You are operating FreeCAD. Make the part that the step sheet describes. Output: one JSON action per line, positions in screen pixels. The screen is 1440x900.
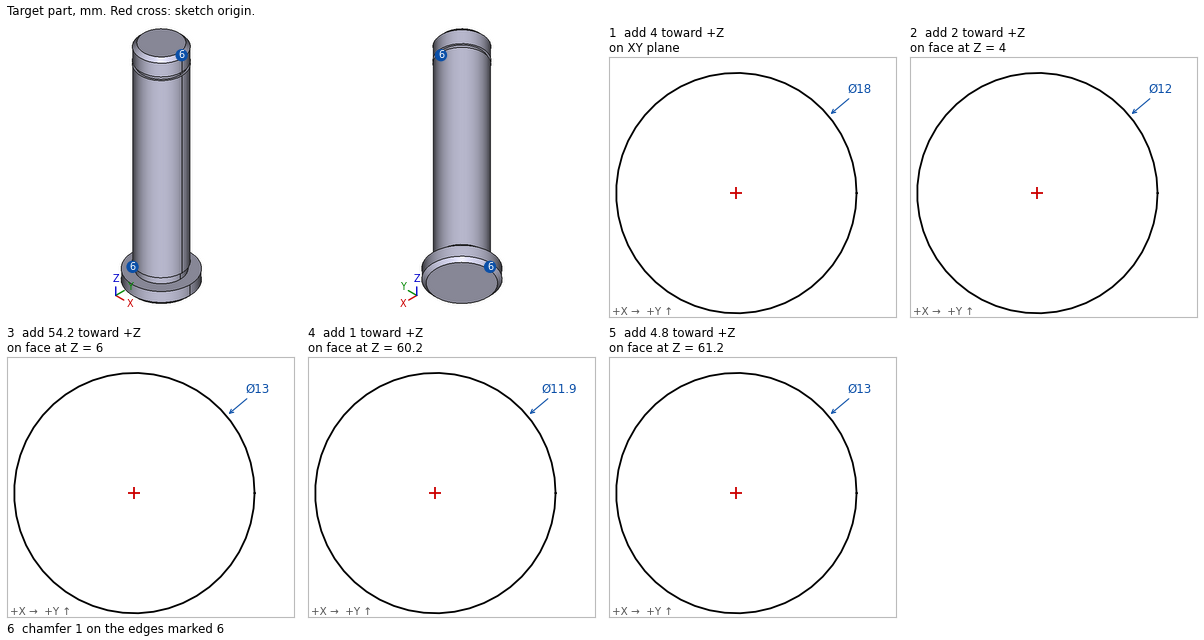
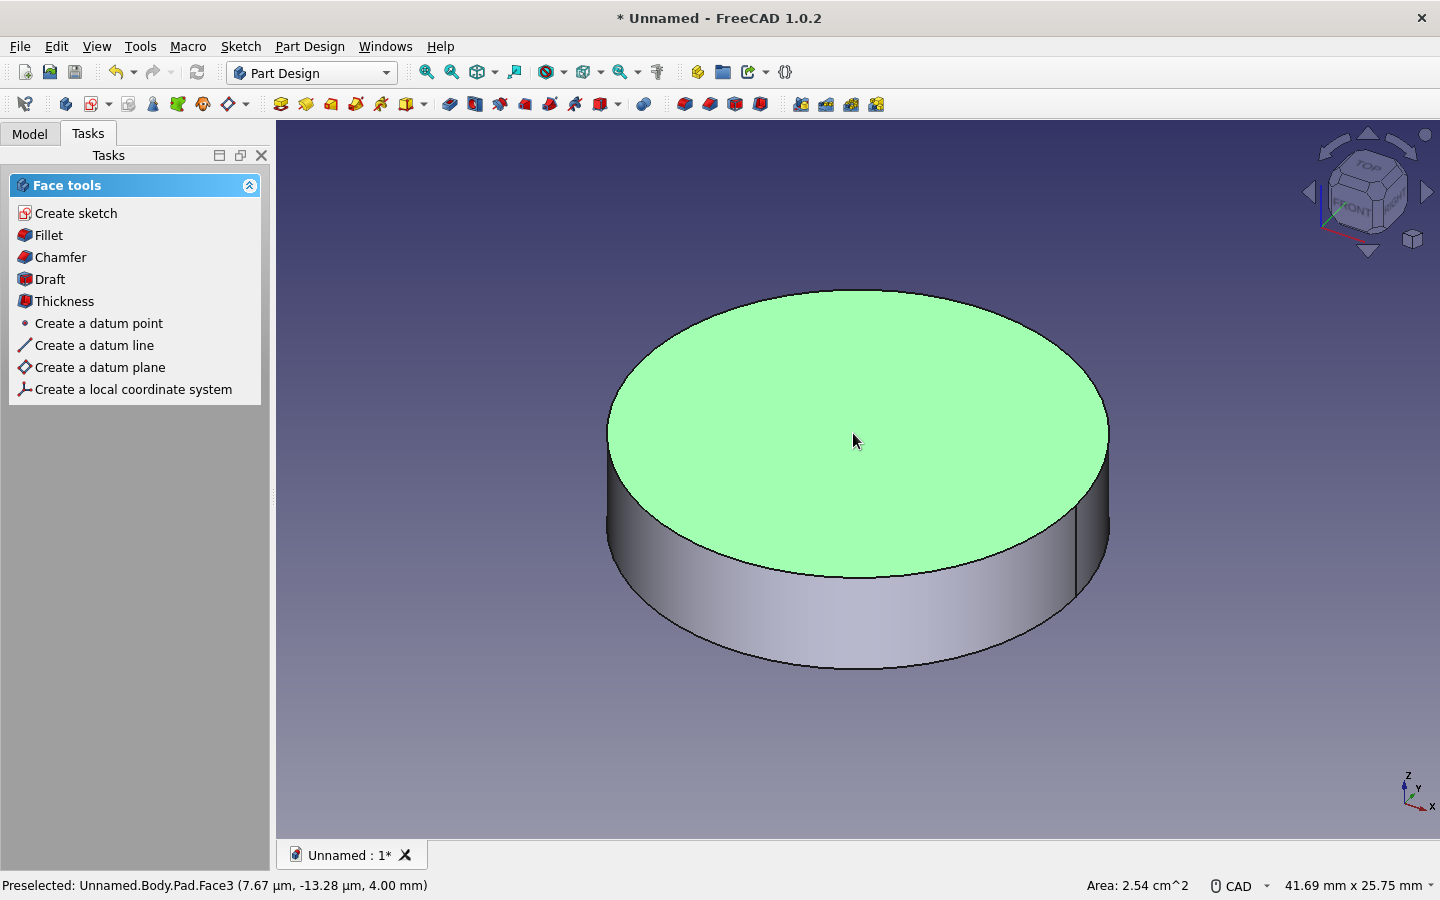
{"action": "left_click", "coordinate": [90, 104]}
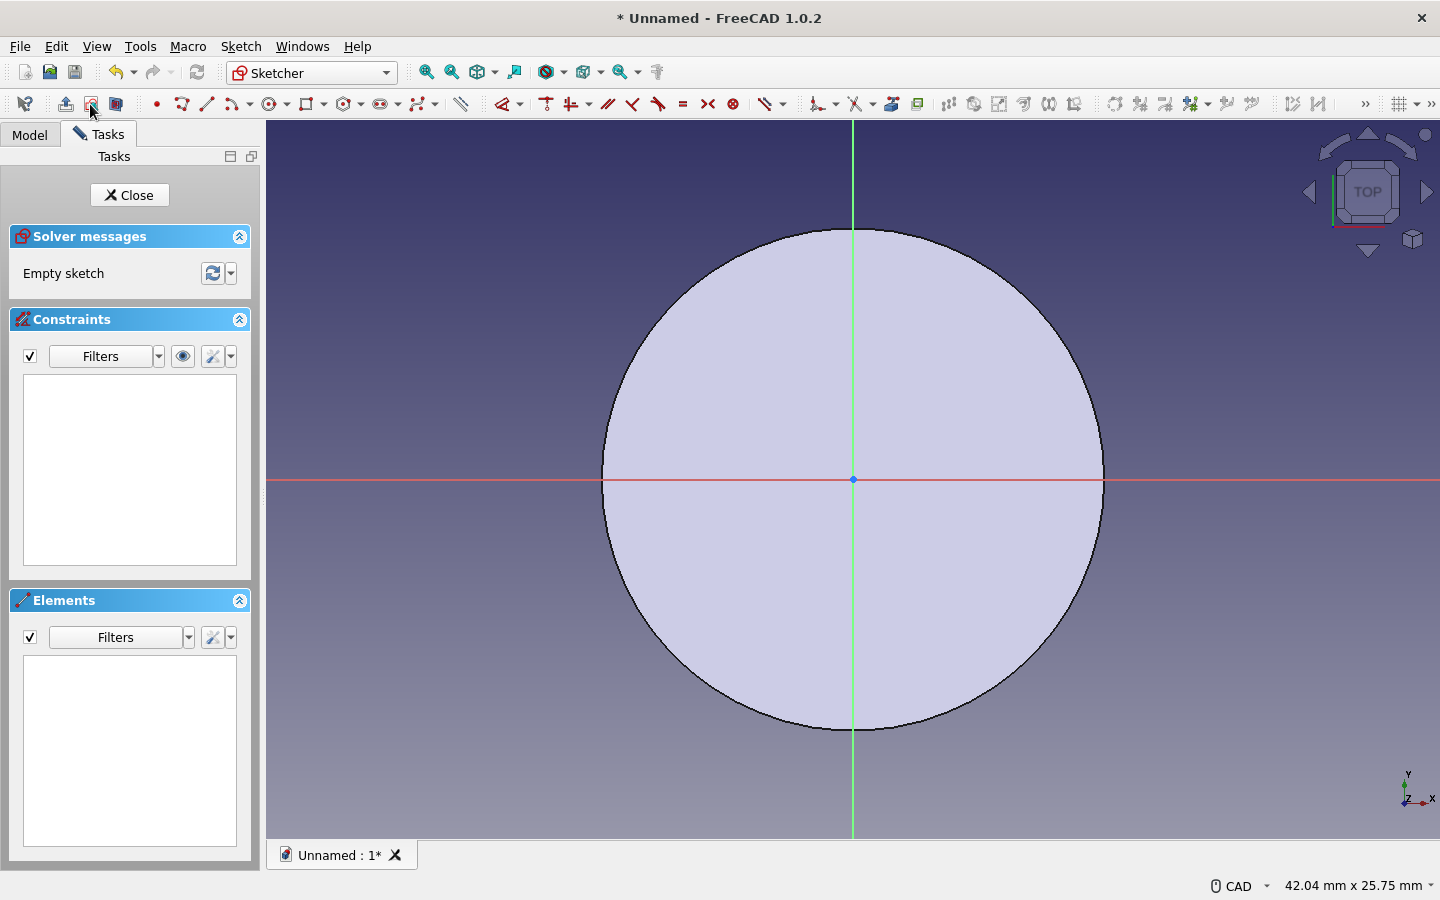
{"action": "scroll", "coordinate": [992, 480], "scroll_direction": "up", "scroll_amount": 2}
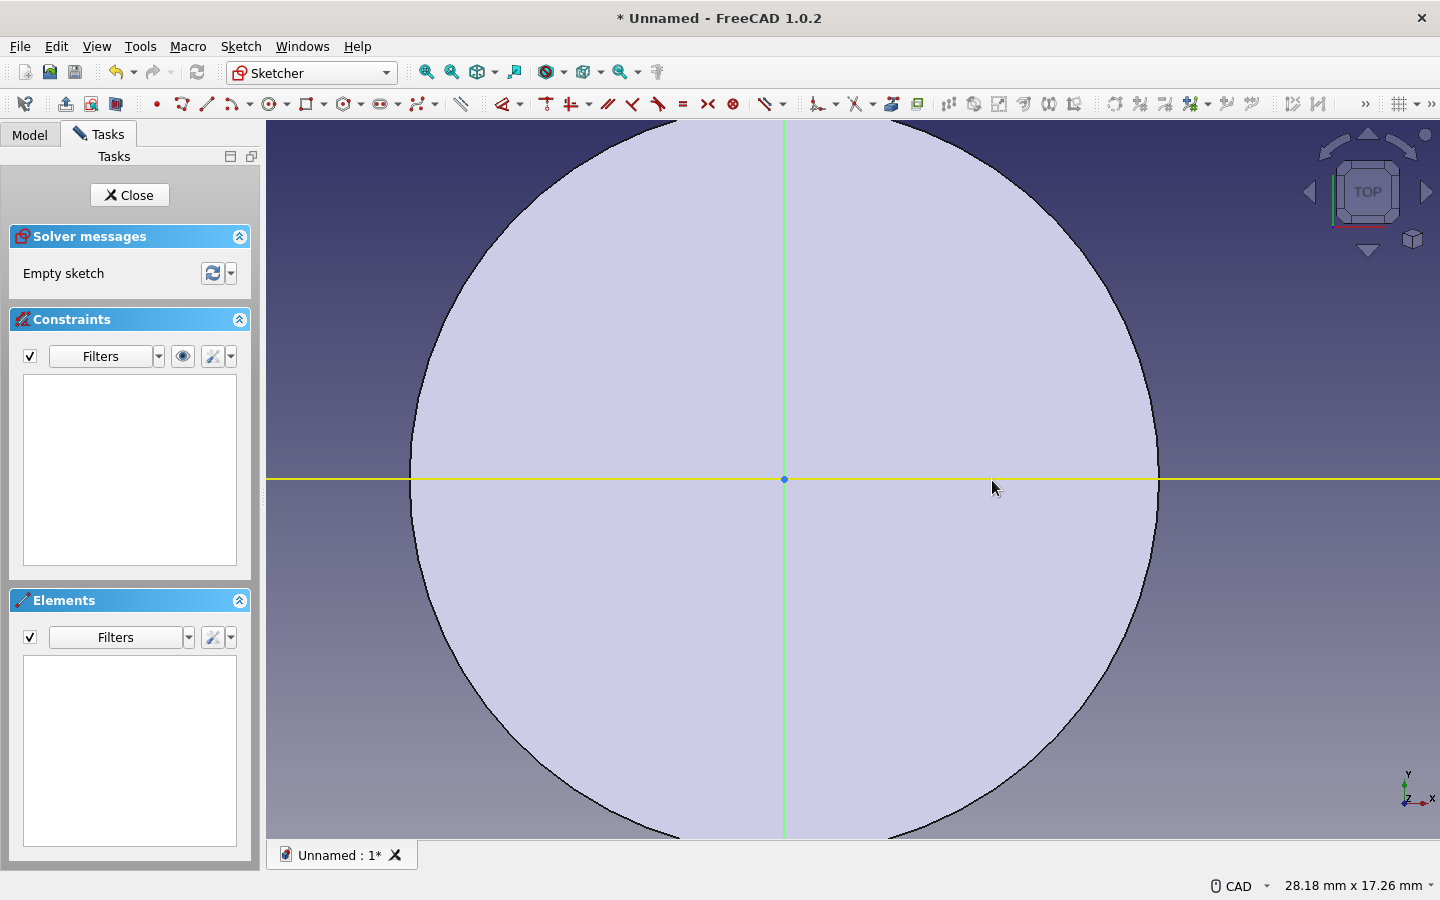
{"action": "left_click", "coordinate": [268, 104]}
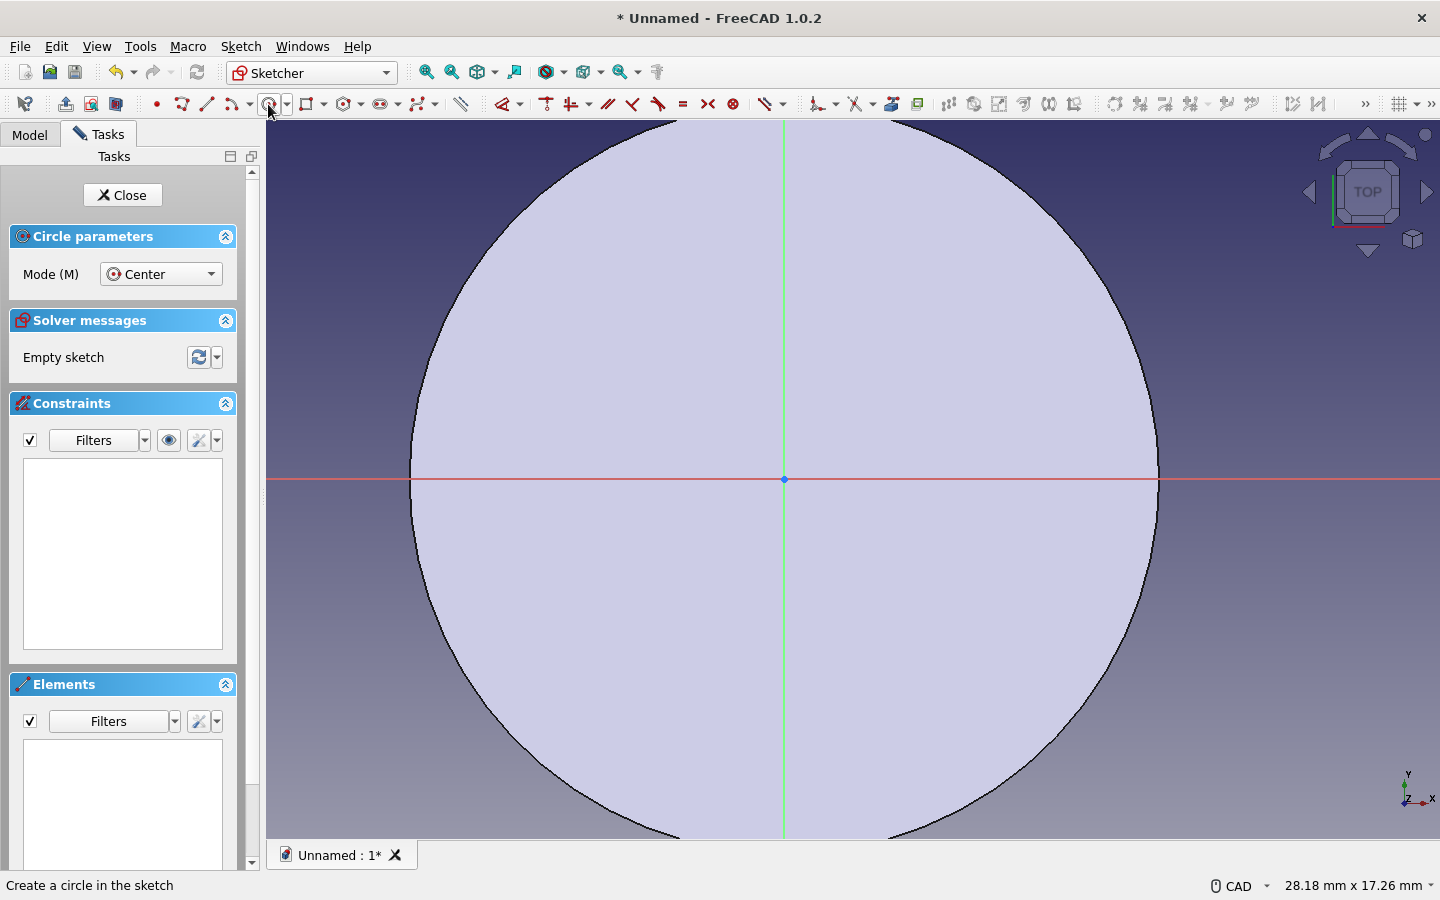
{"action": "left_click", "coordinate": [784, 479]}
{"action": "left_click", "coordinate": [961, 302]}
{"action": "key", "text": "Escape"}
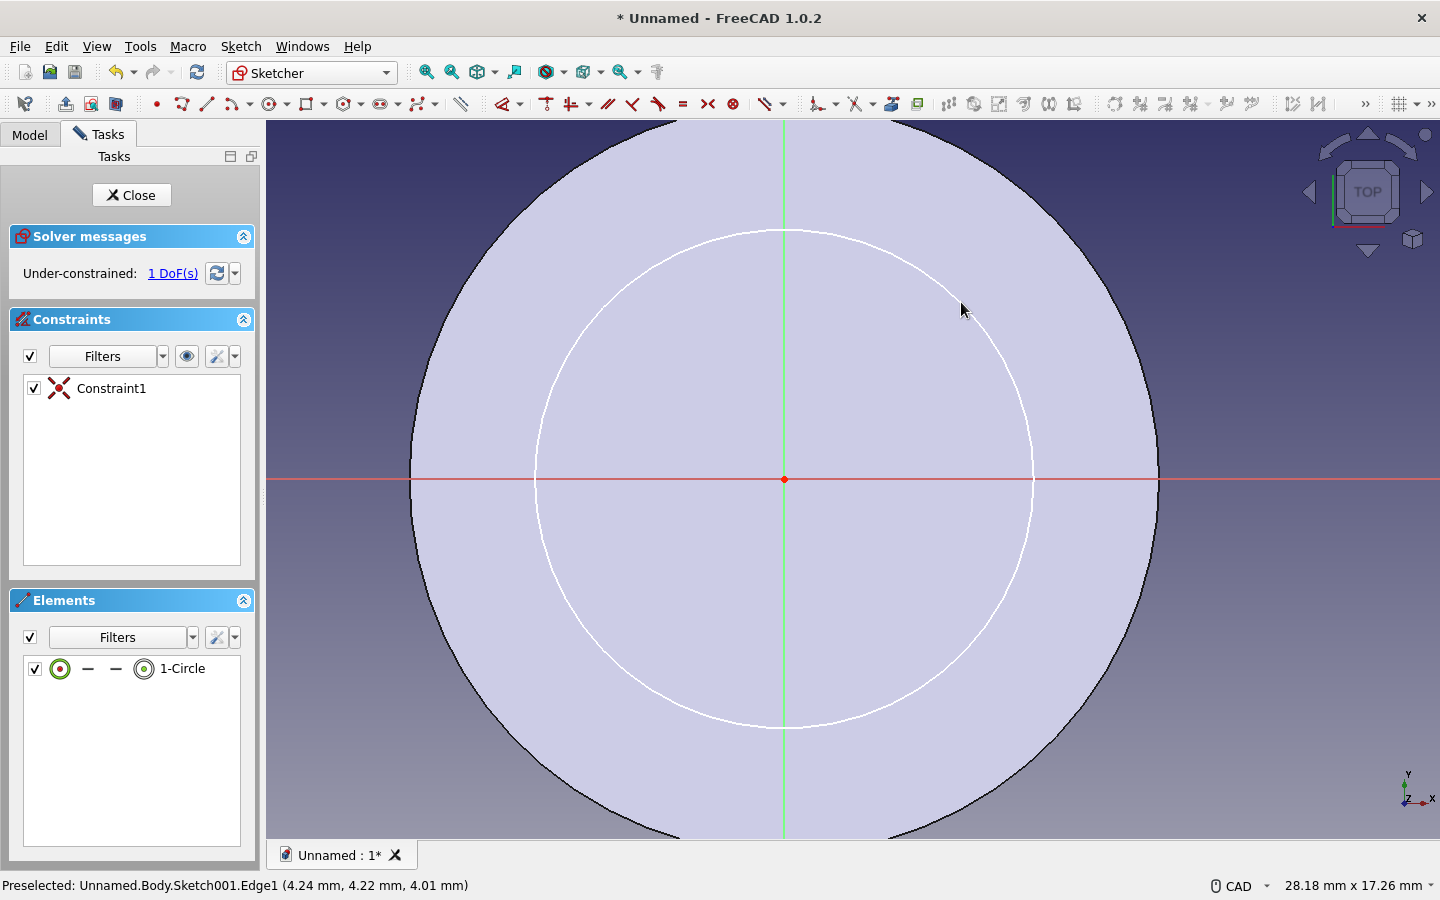
{"action": "left_click", "coordinate": [502, 104]}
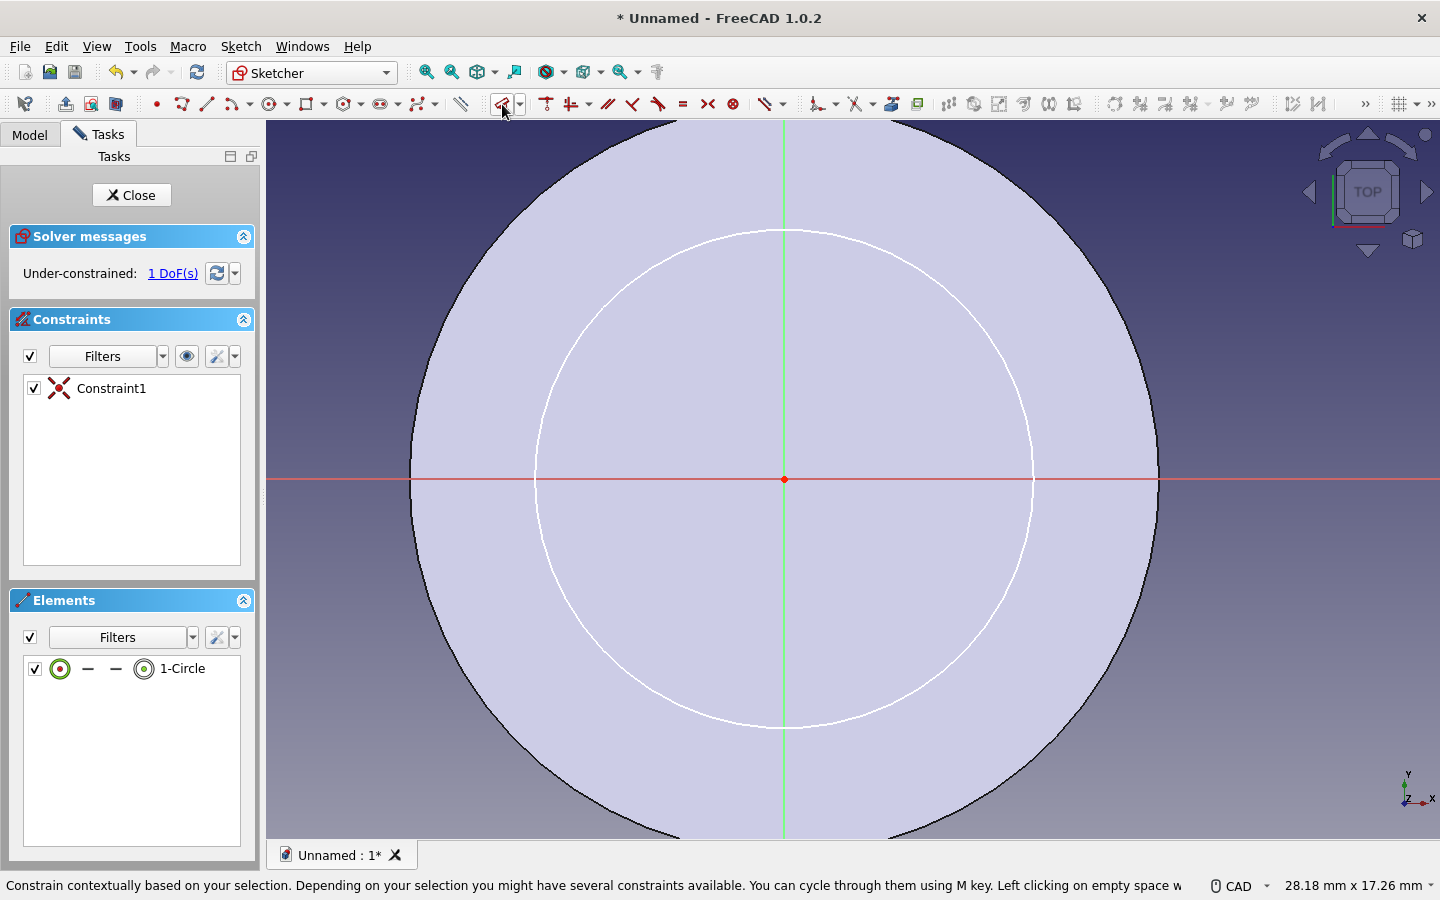
{"action": "left_click", "coordinate": [960, 302]}
{"action": "left_click", "coordinate": [983, 279]}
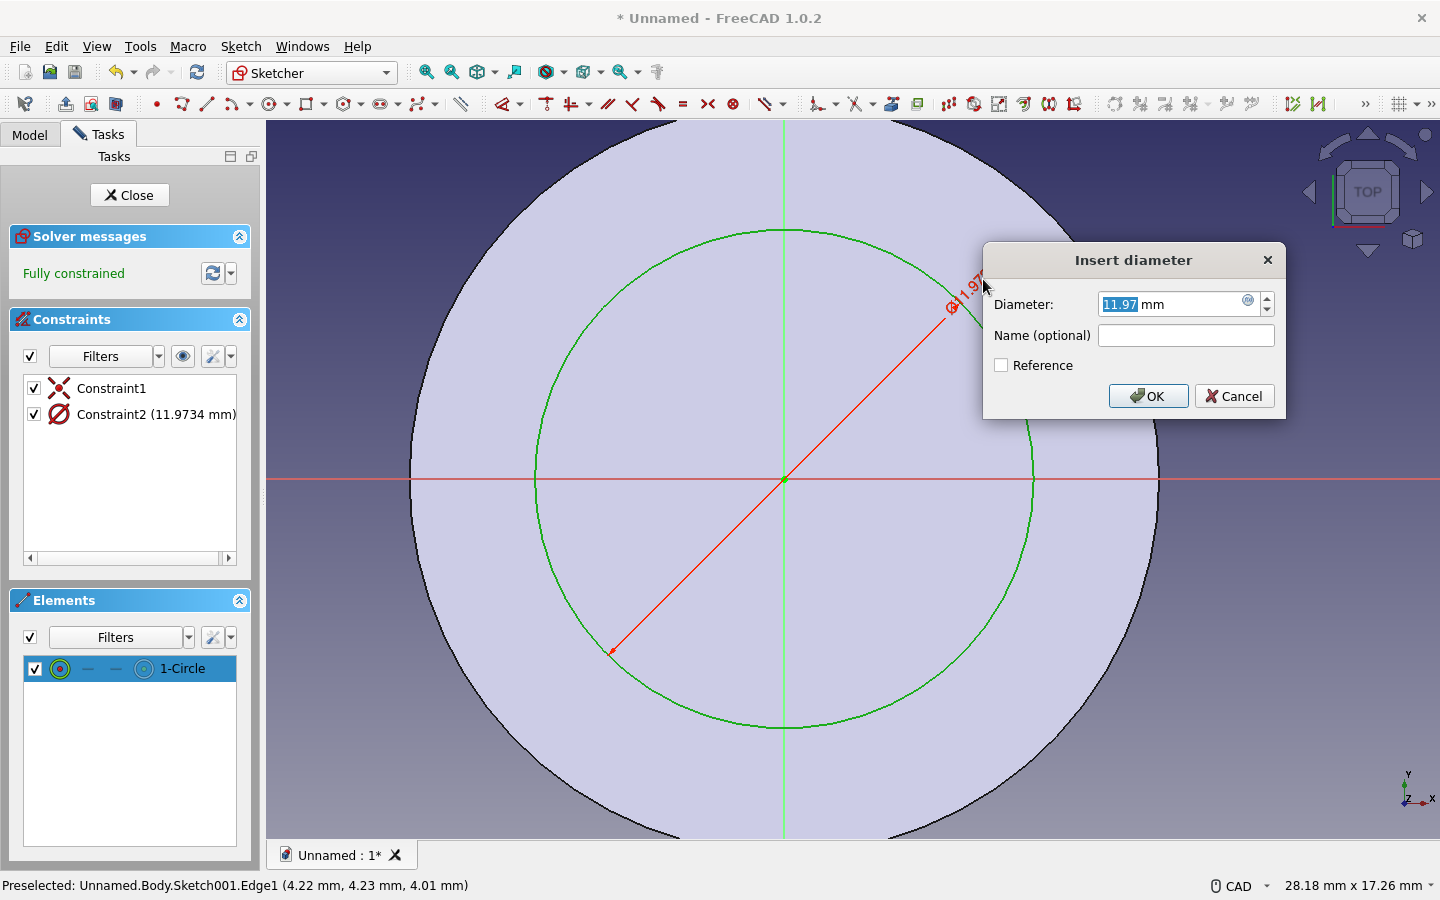
{"action": "type", "text": "12"}
{"action": "key", "text": "Return"}
{"action": "key", "text": "Escape"}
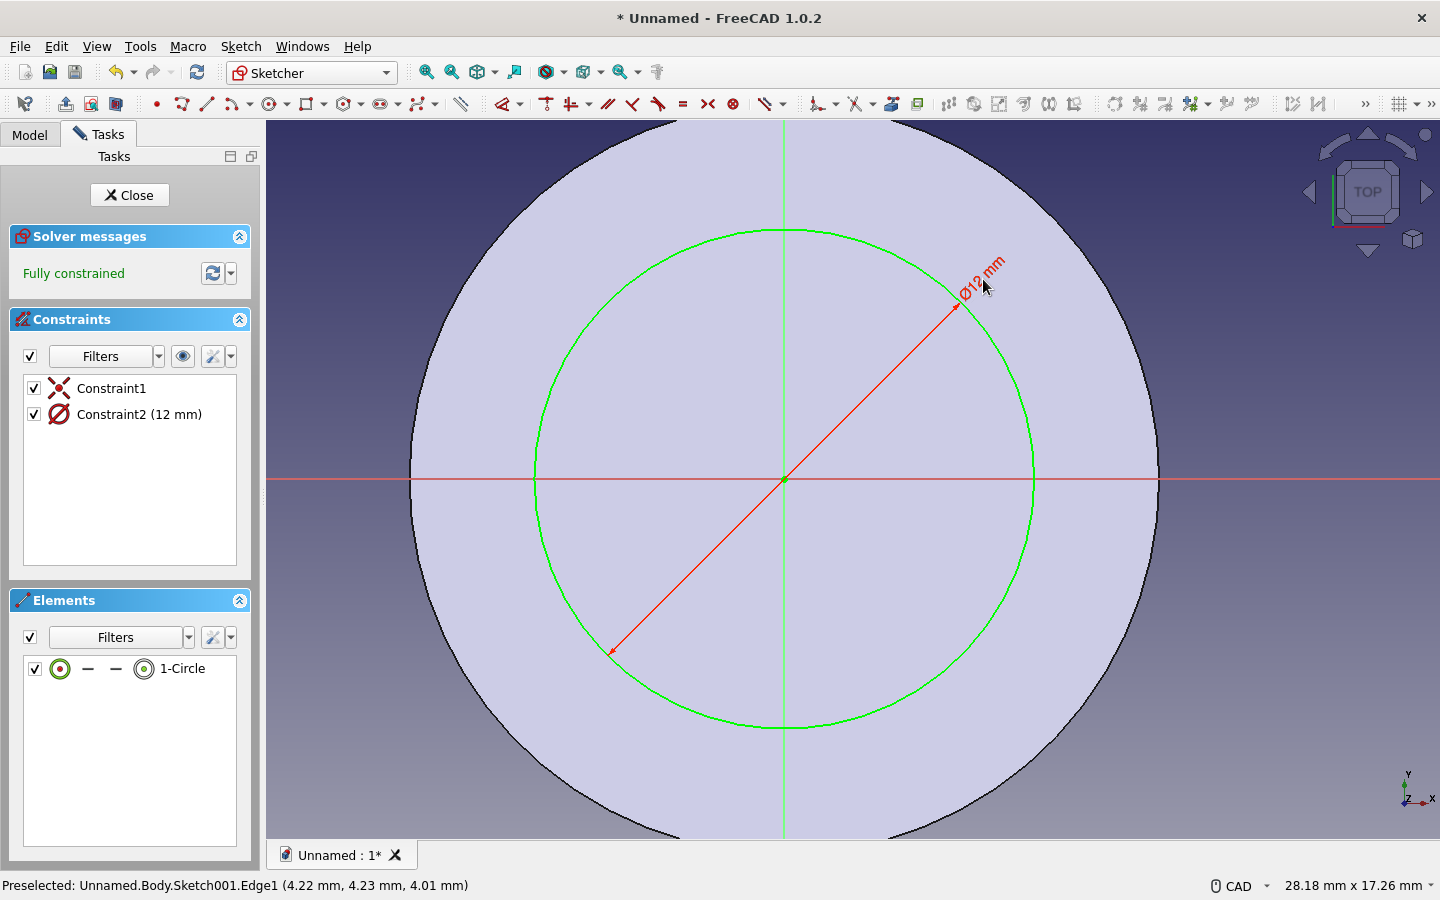
{"action": "left_click", "coordinate": [130, 195]}